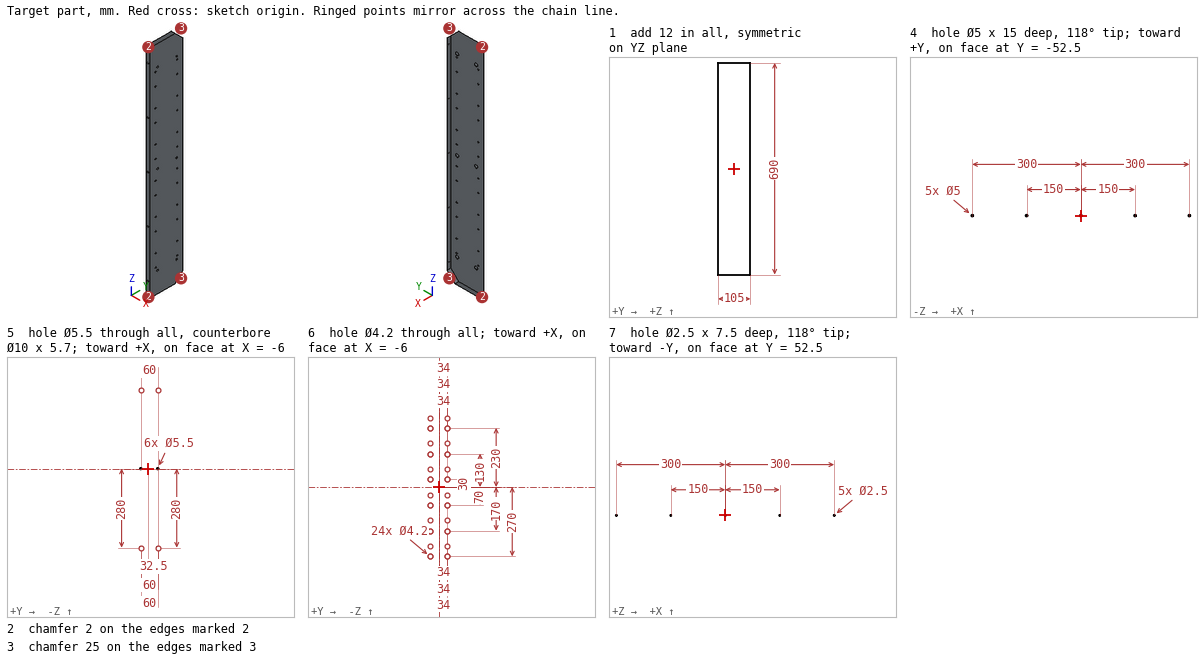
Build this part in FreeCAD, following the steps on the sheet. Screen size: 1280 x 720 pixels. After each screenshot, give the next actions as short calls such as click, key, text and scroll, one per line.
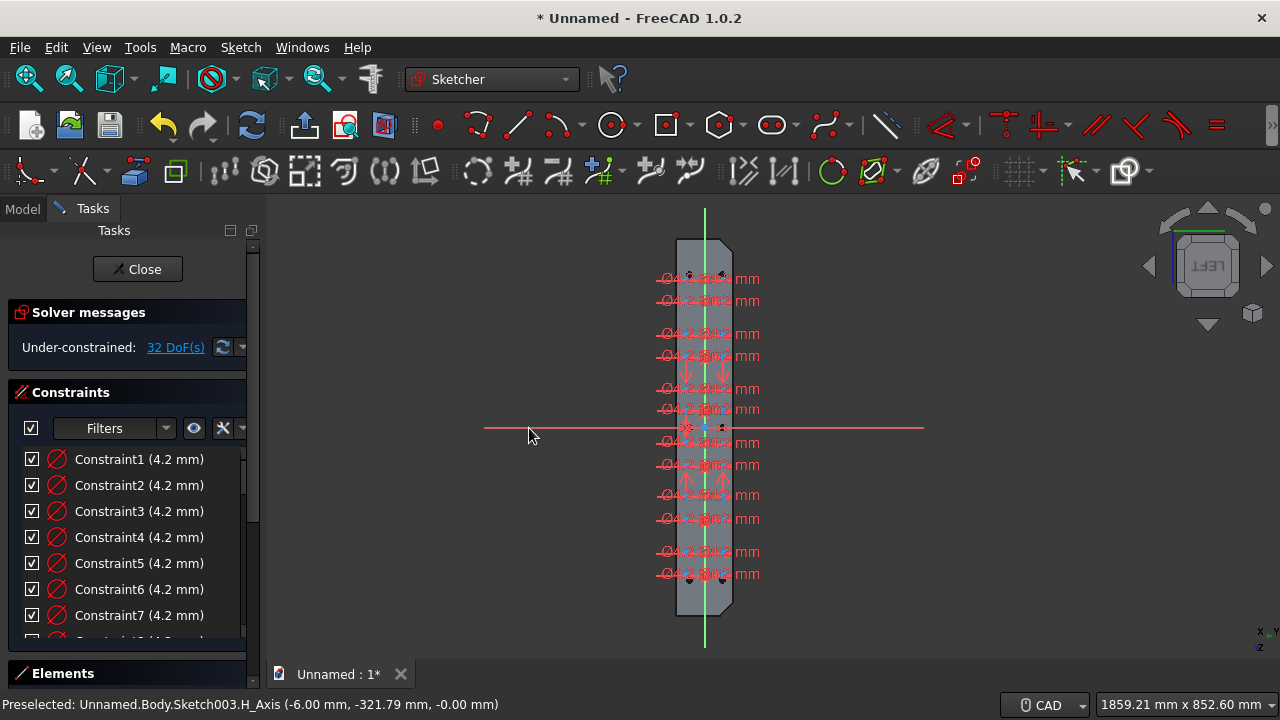
click(723, 411)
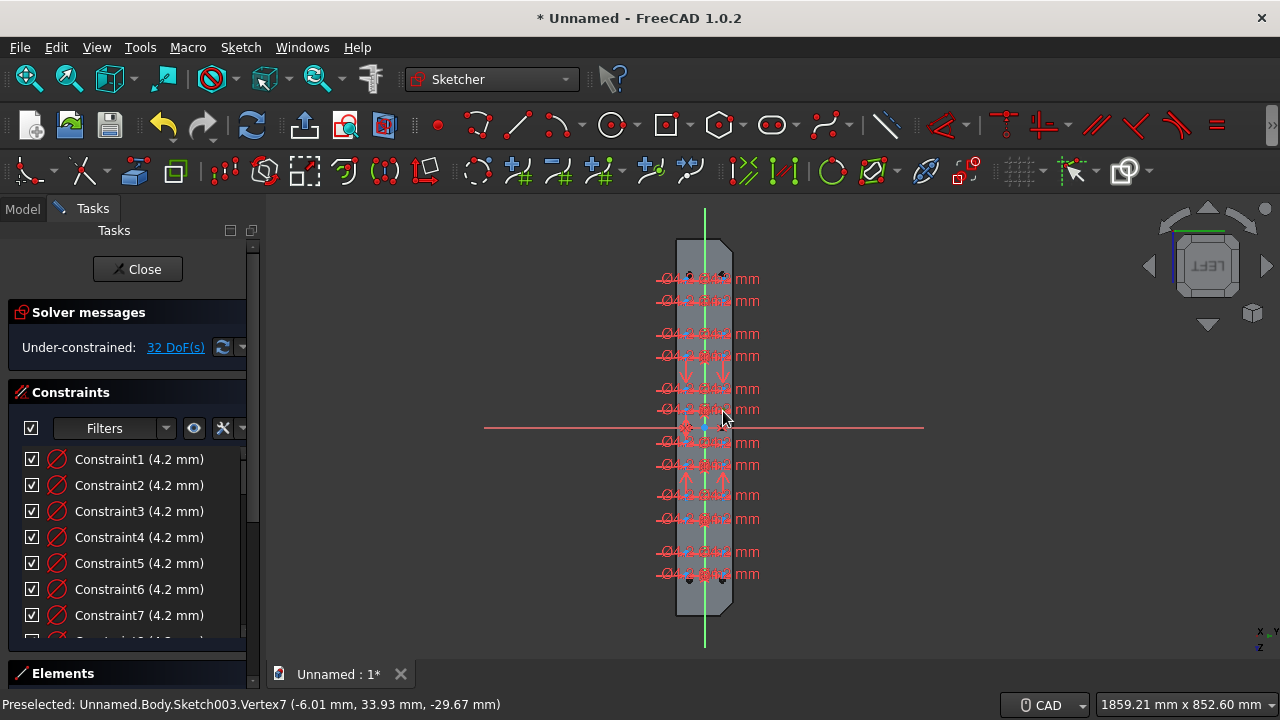
click(723, 445)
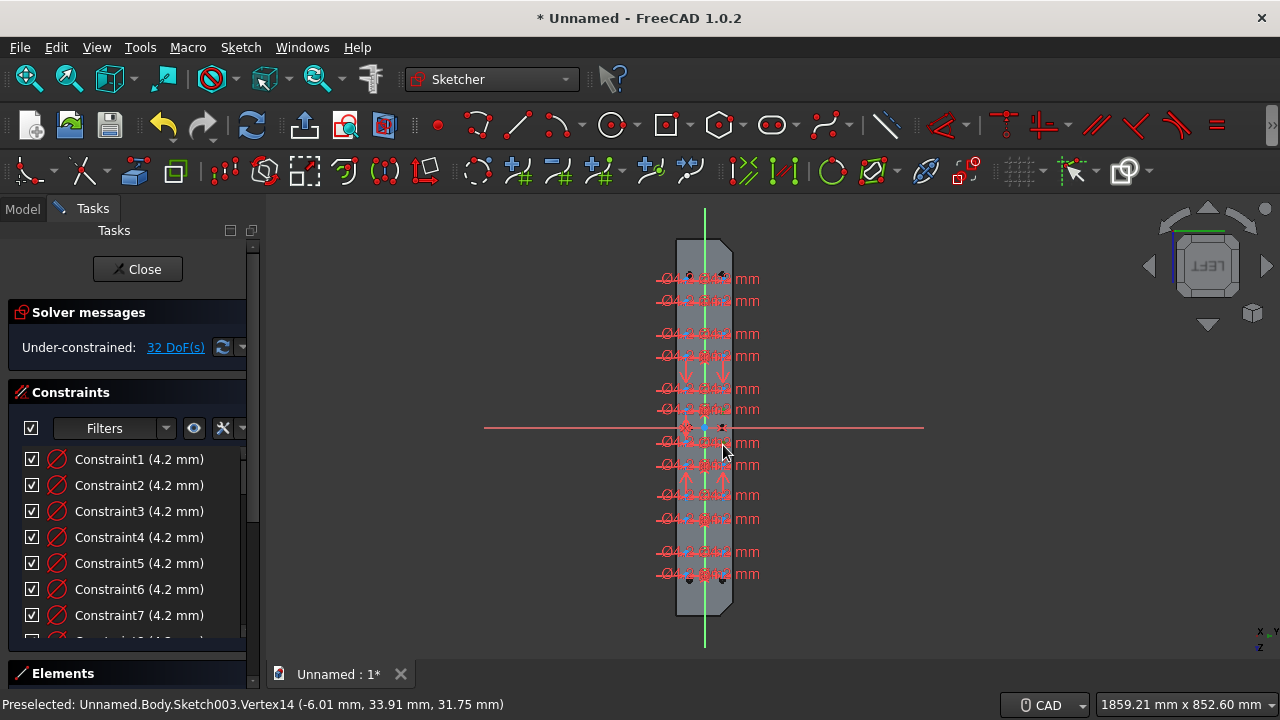
click(529, 428)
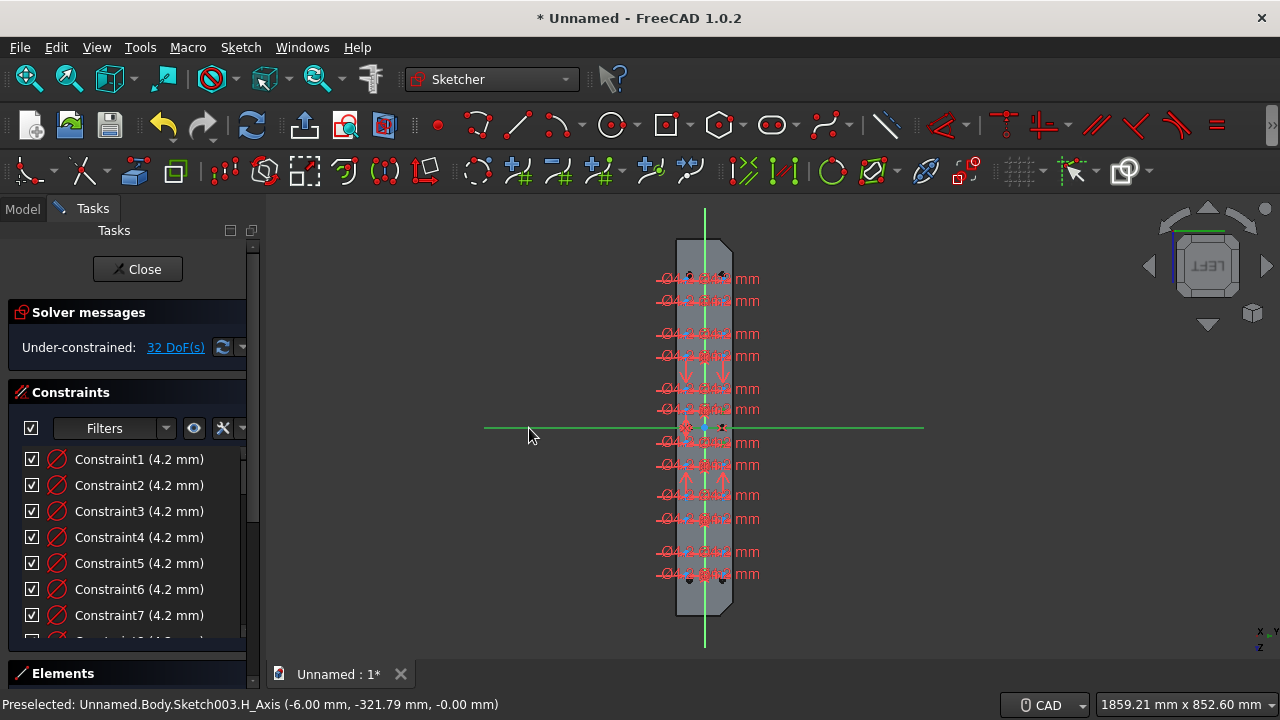
key(s)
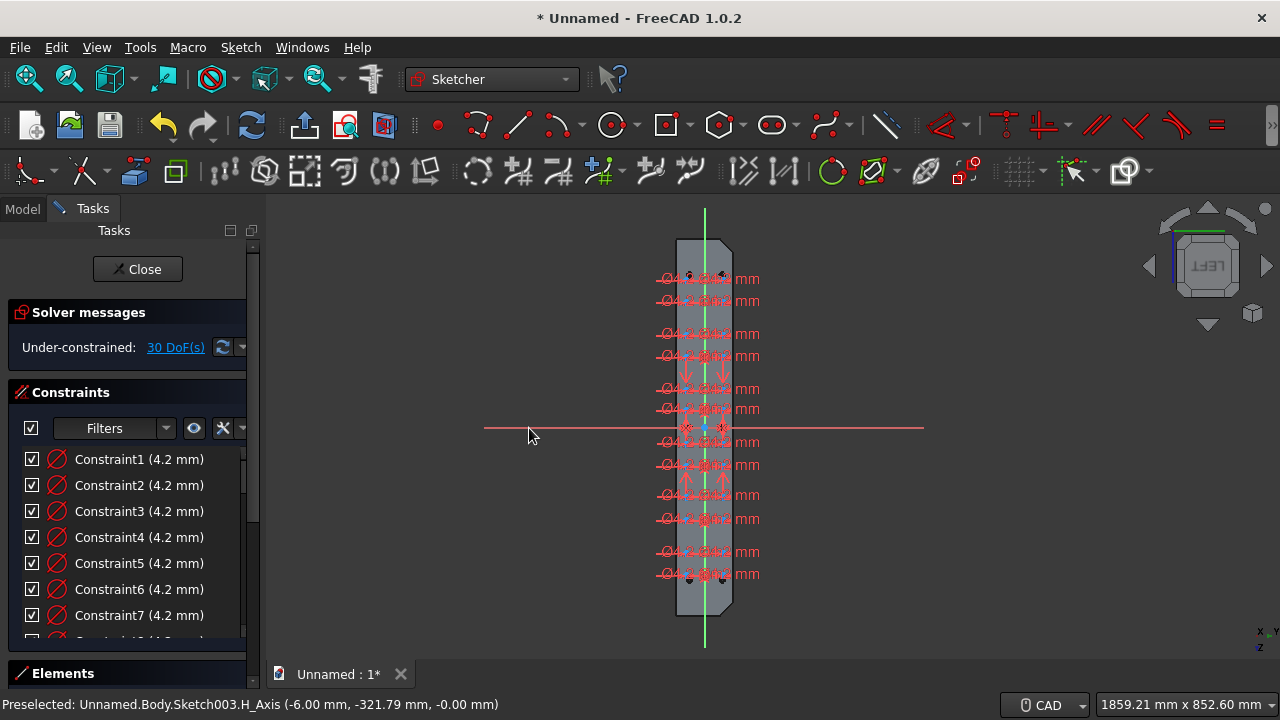
click(686, 467)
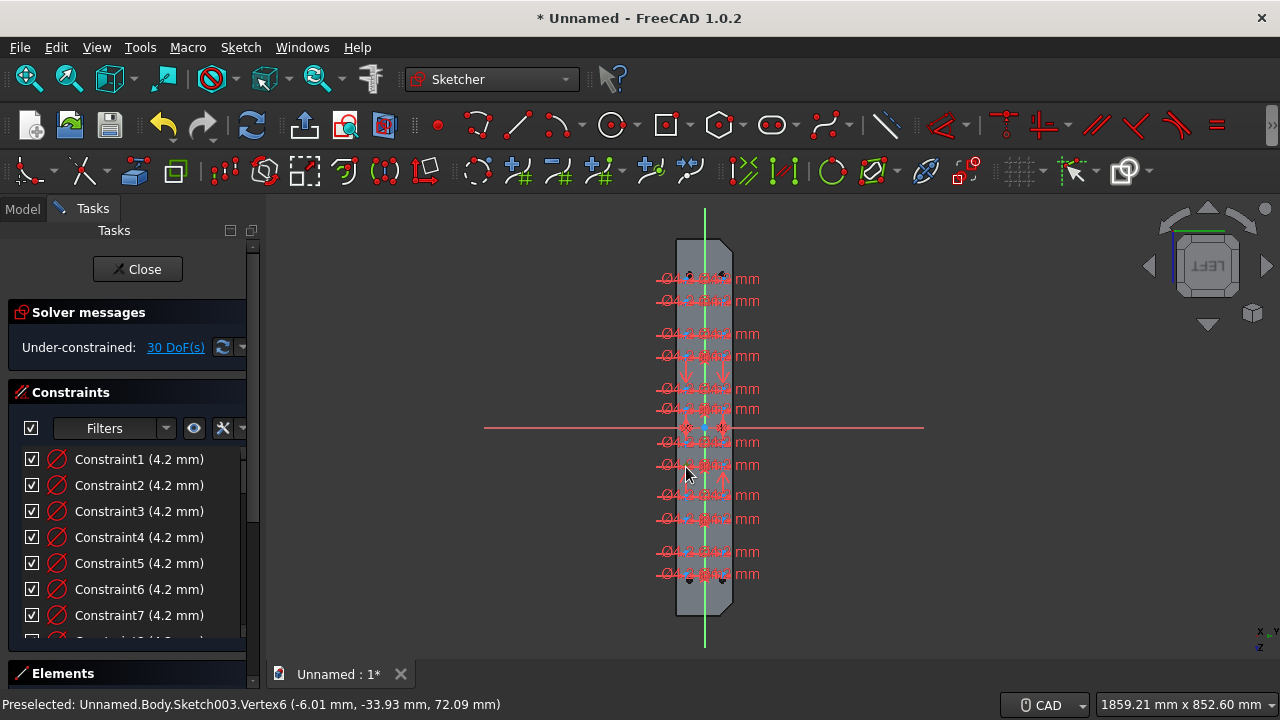
click(686, 391)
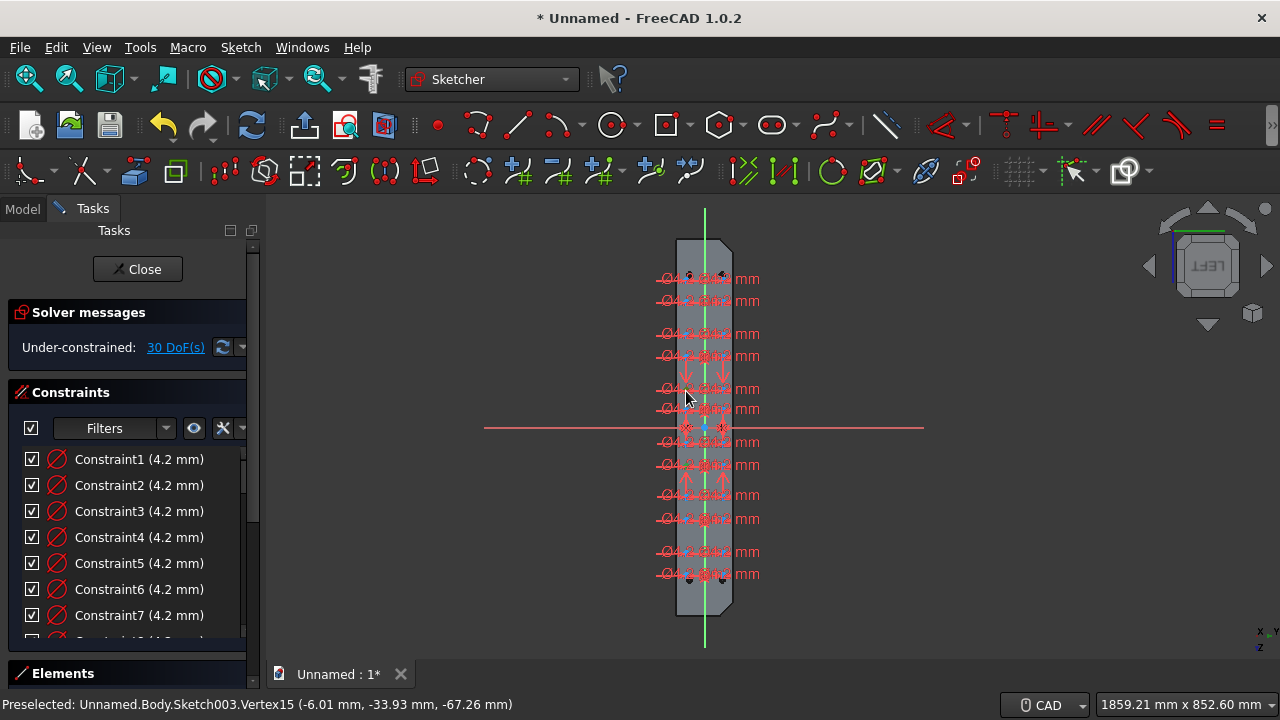
click(529, 428)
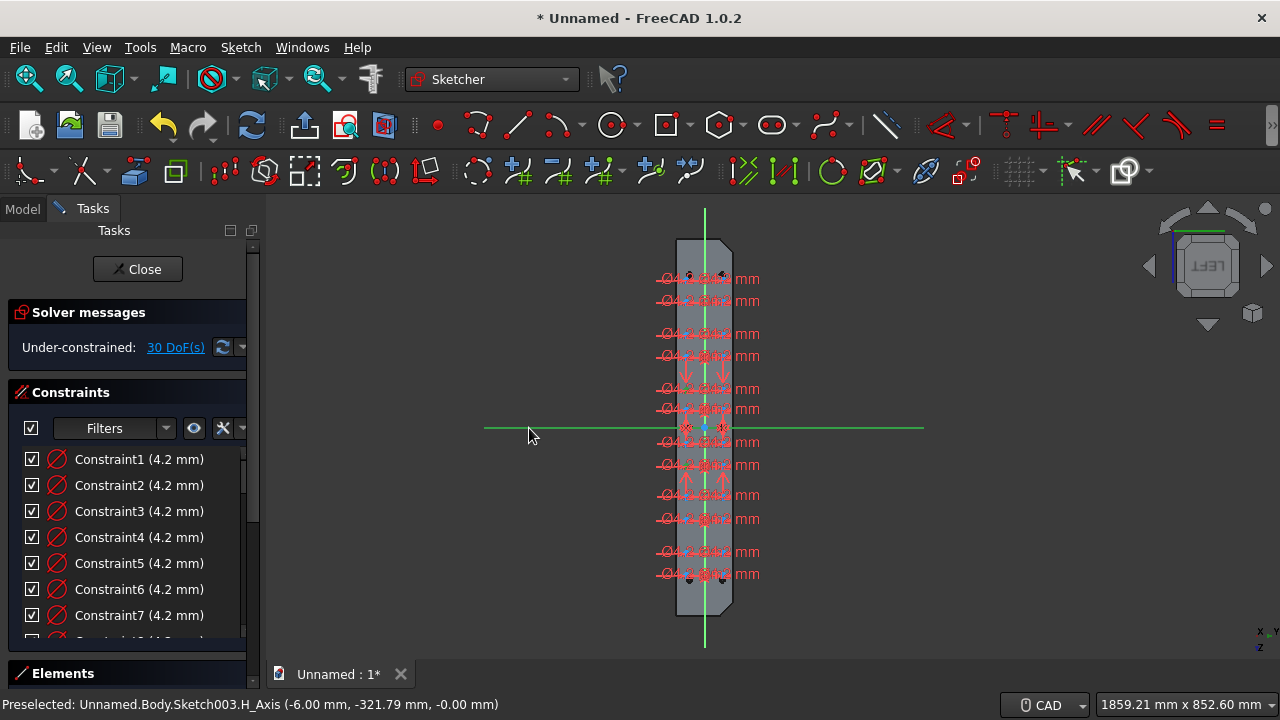
key(s)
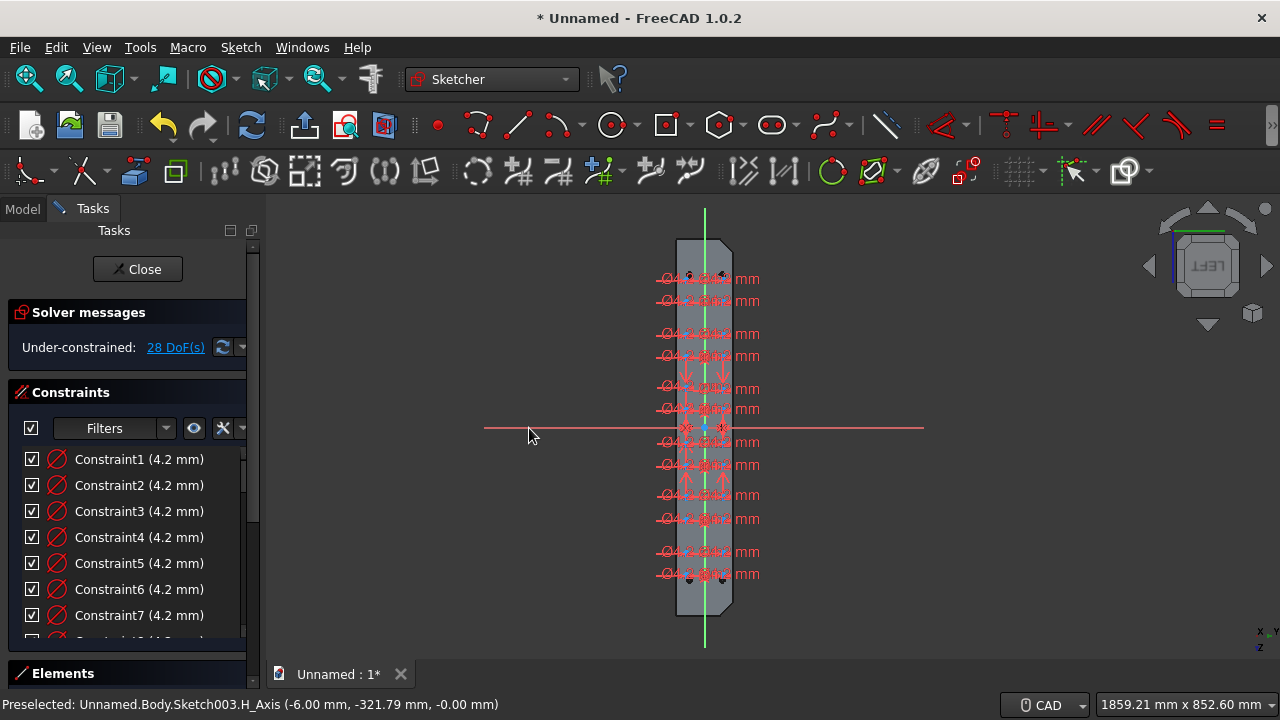
click(723, 467)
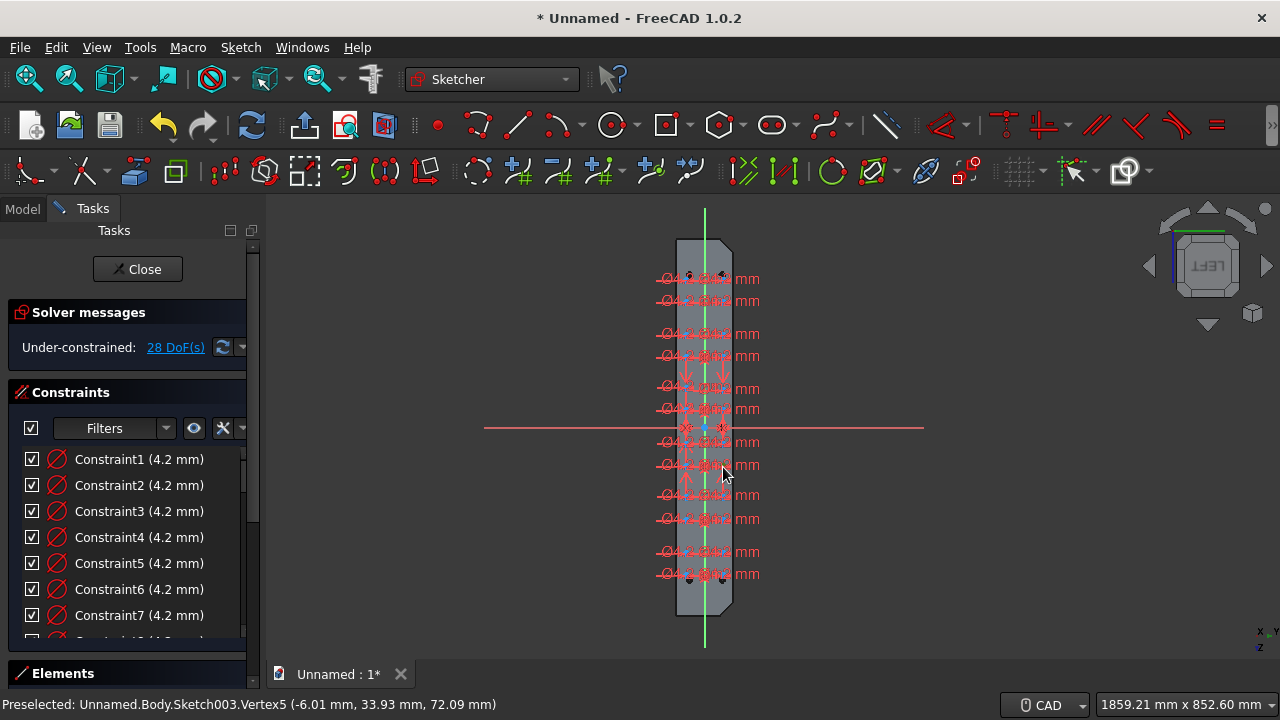
click(723, 391)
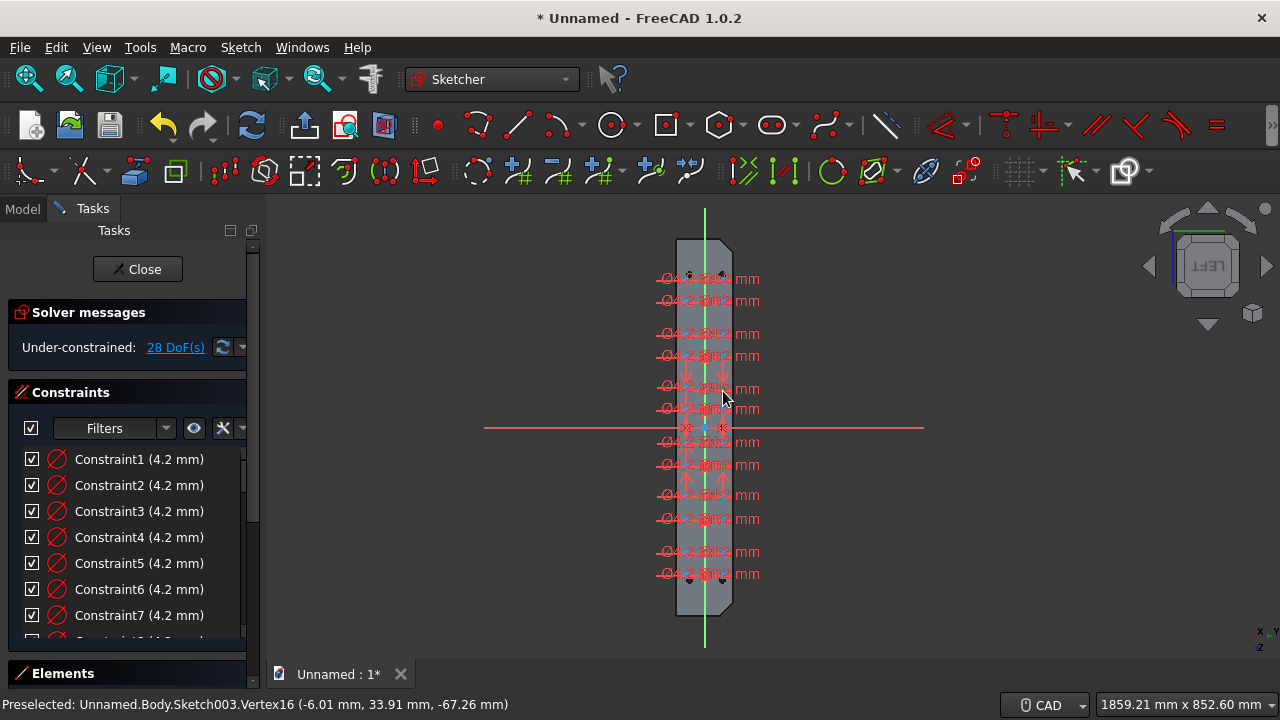
click(529, 428)